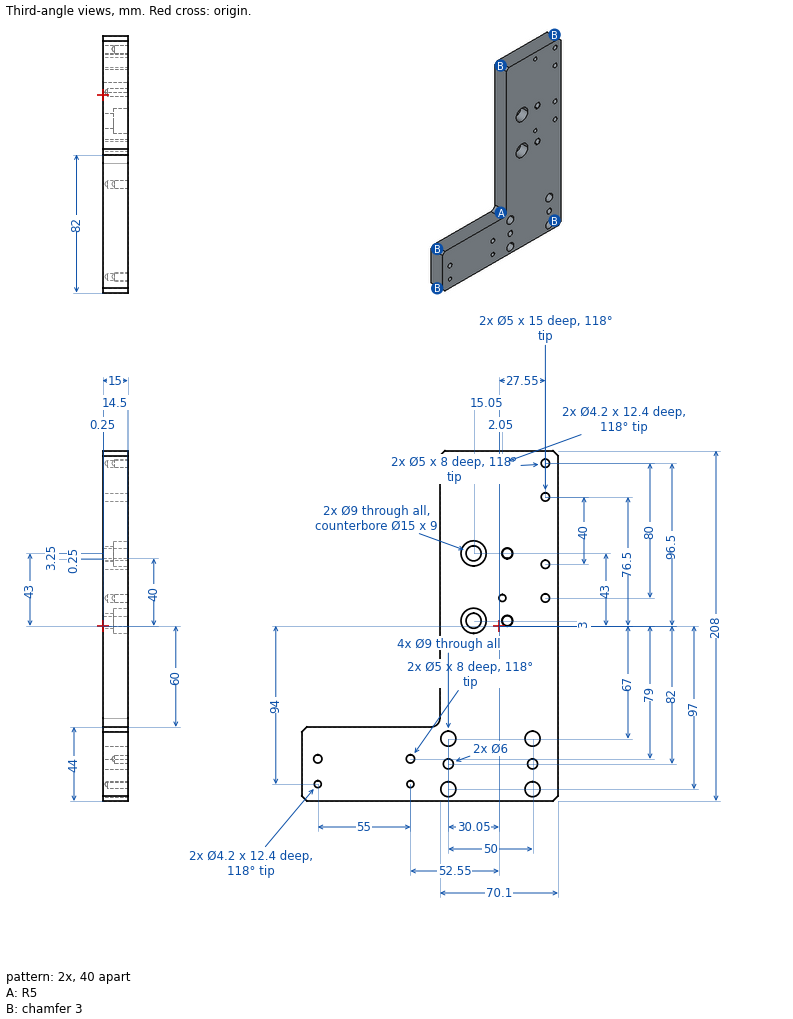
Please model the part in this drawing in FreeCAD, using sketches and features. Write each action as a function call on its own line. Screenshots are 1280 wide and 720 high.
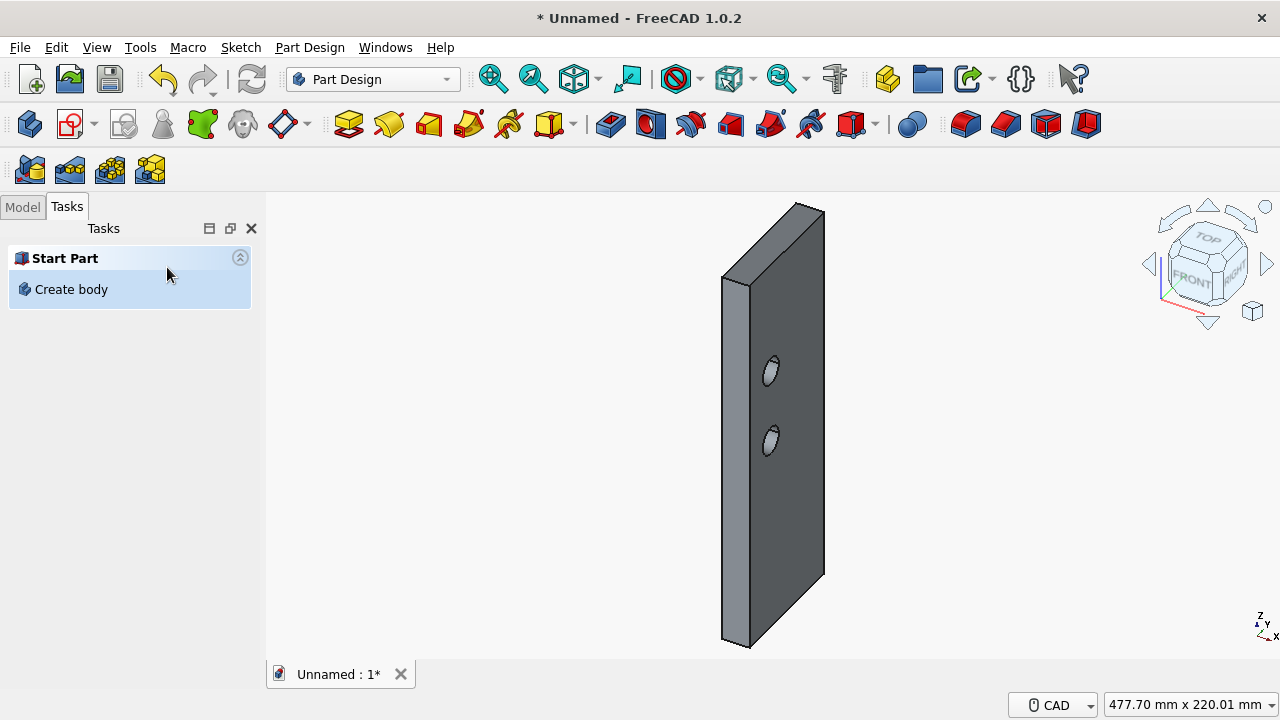
click(23, 206)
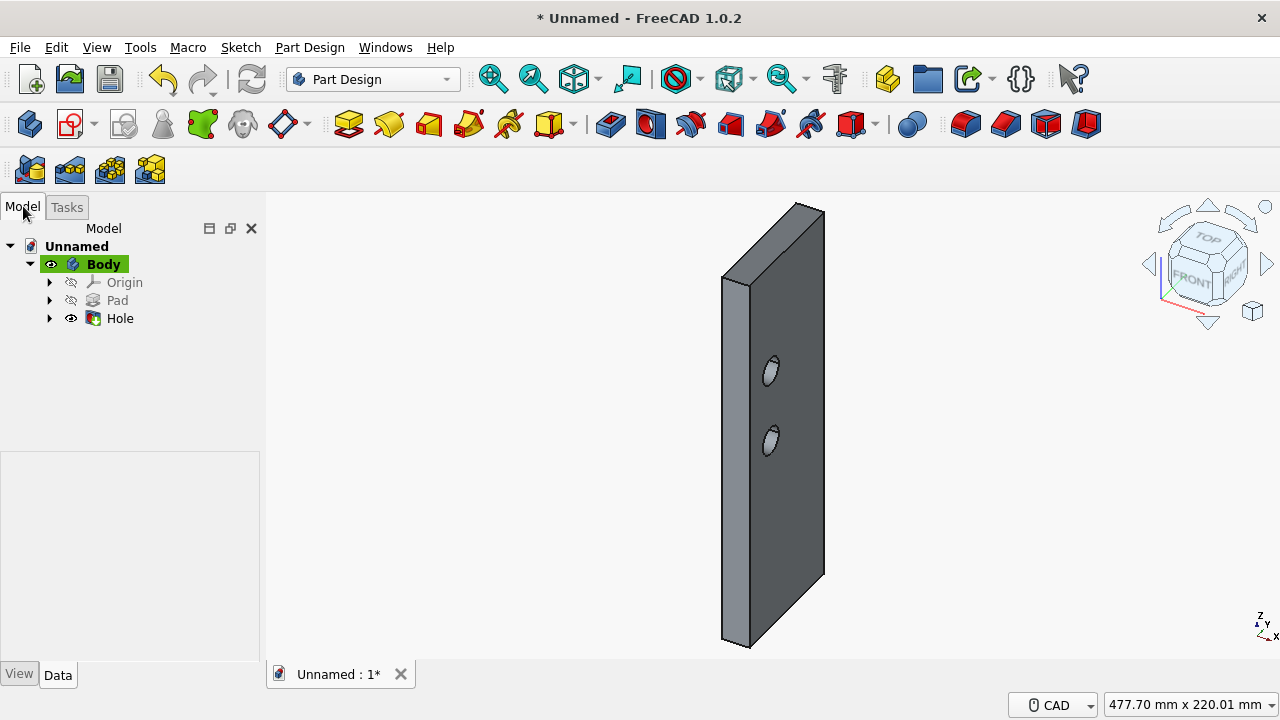
click(50, 282)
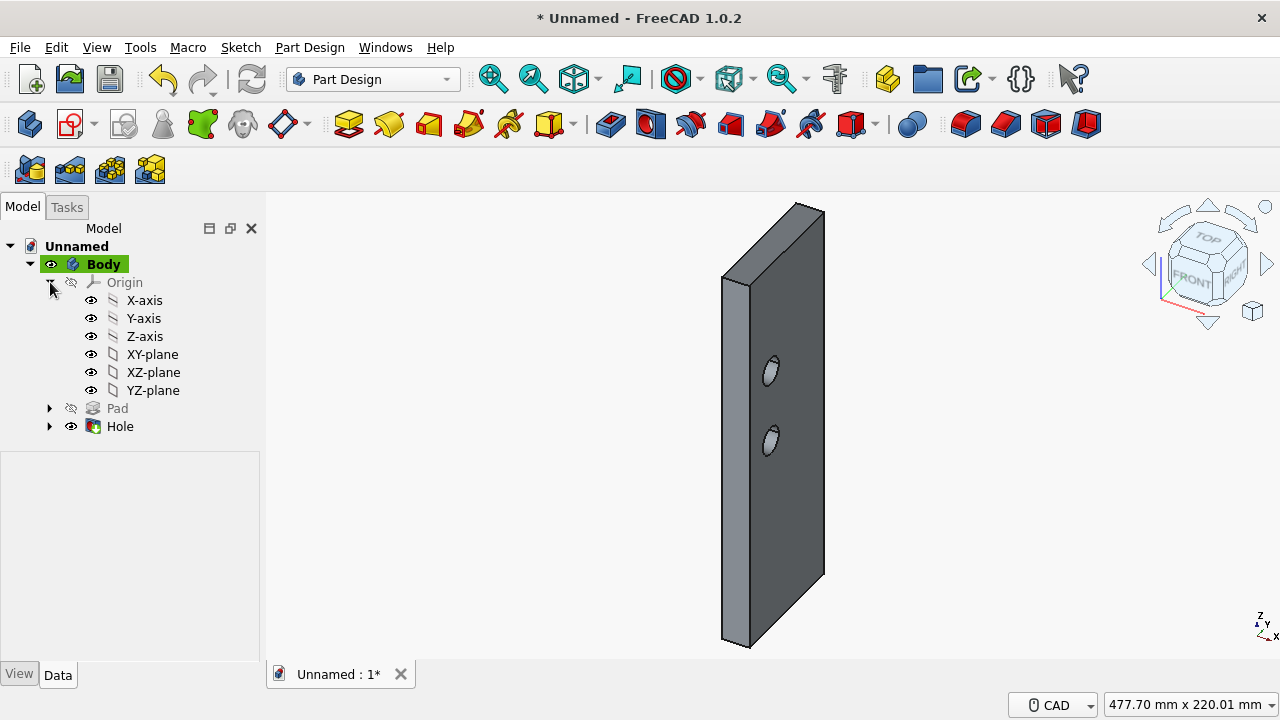
click(136, 372)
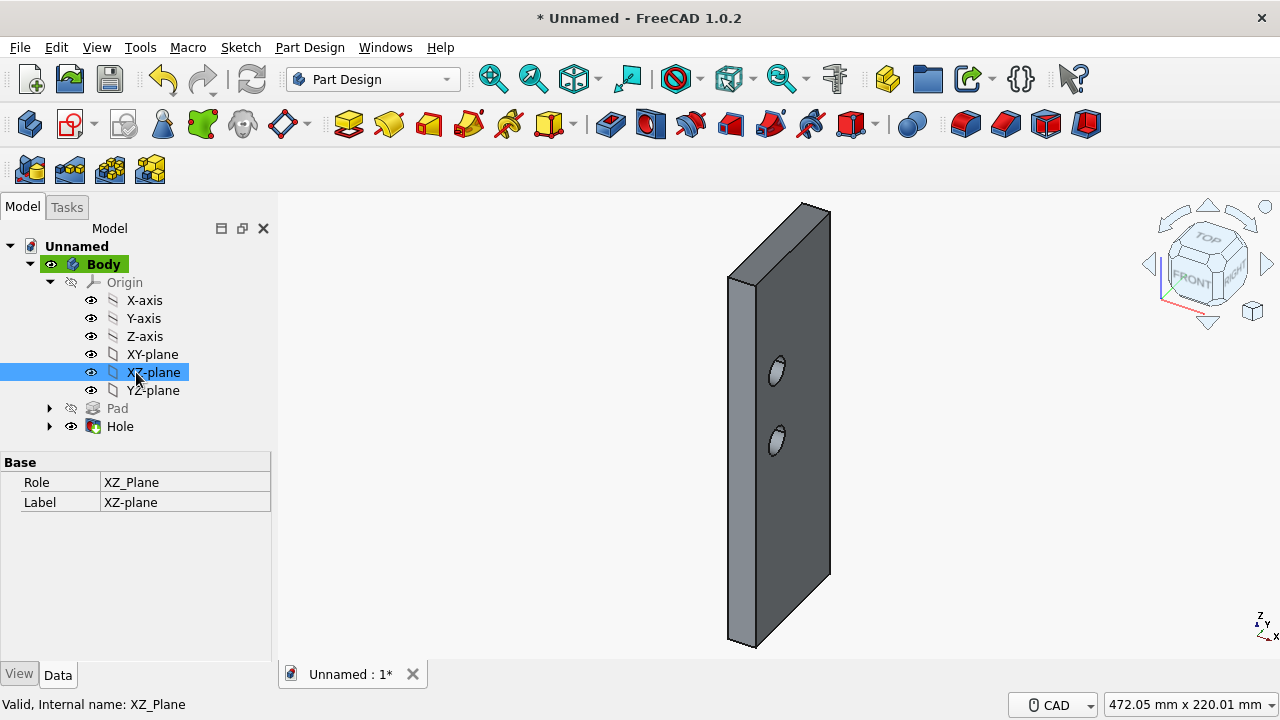
click(284, 124)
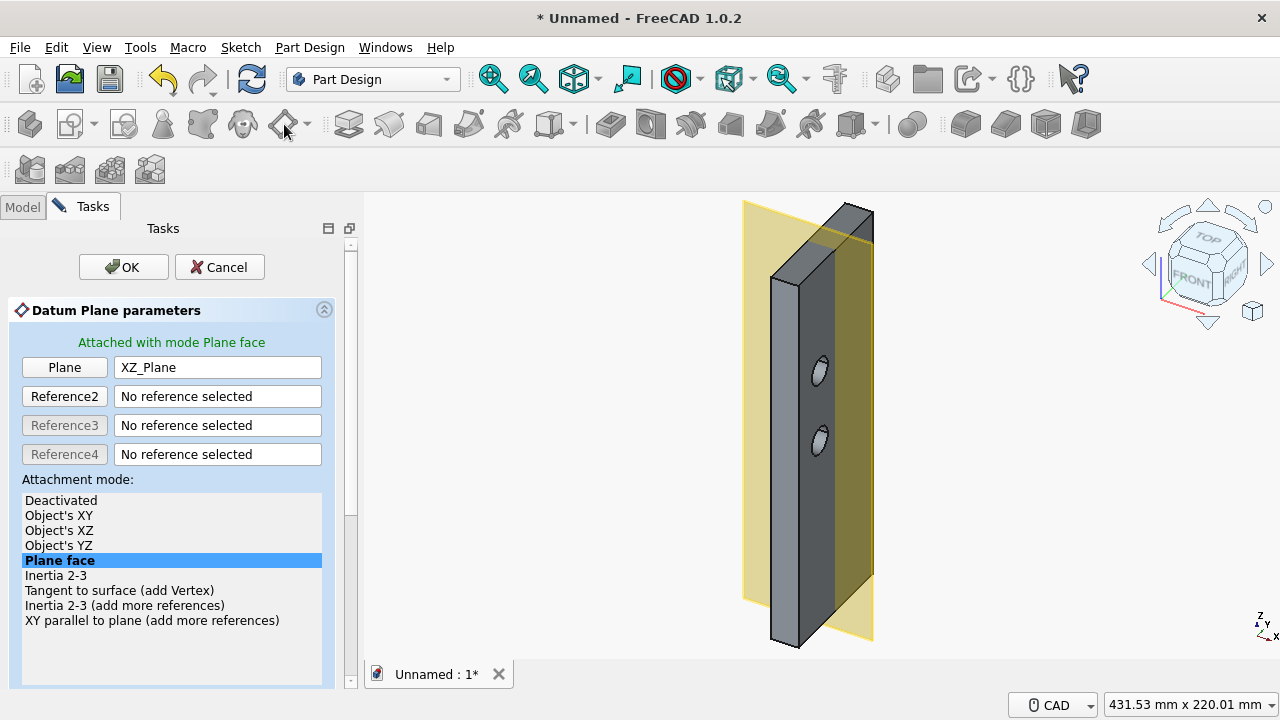
scroll(351, 463, down, 3)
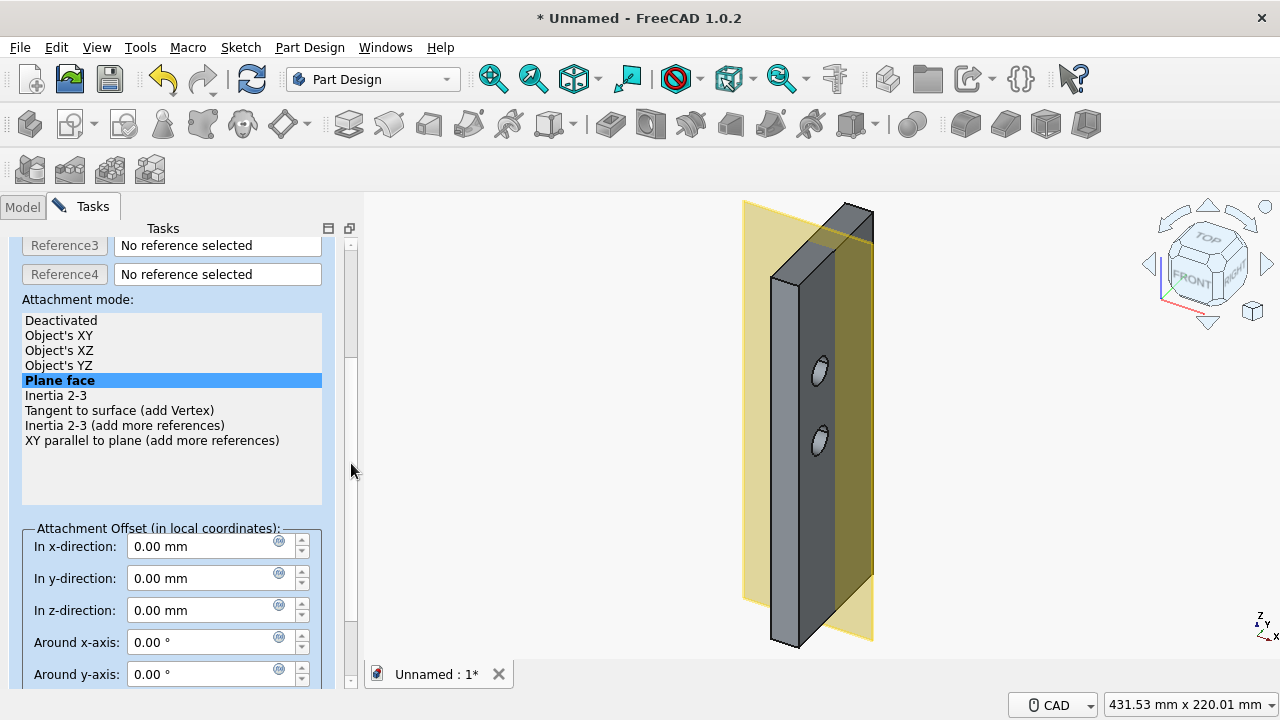
triple_click(210, 610)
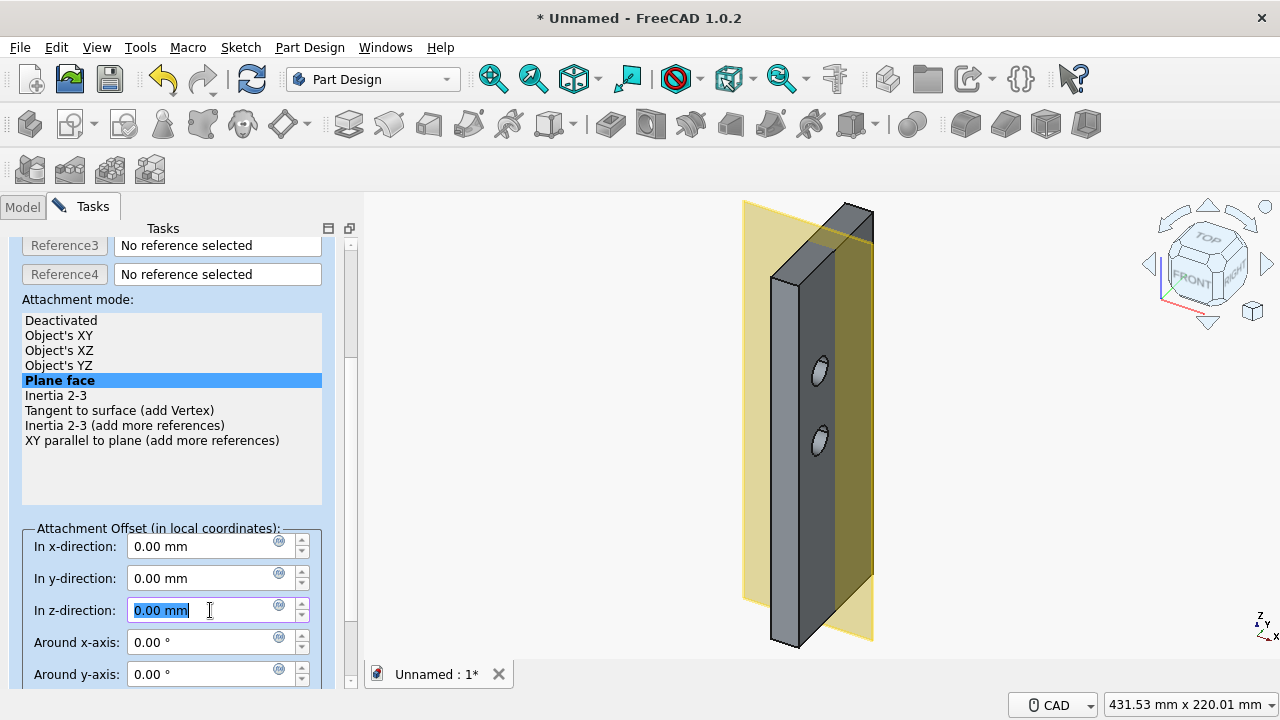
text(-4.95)
key(Tab)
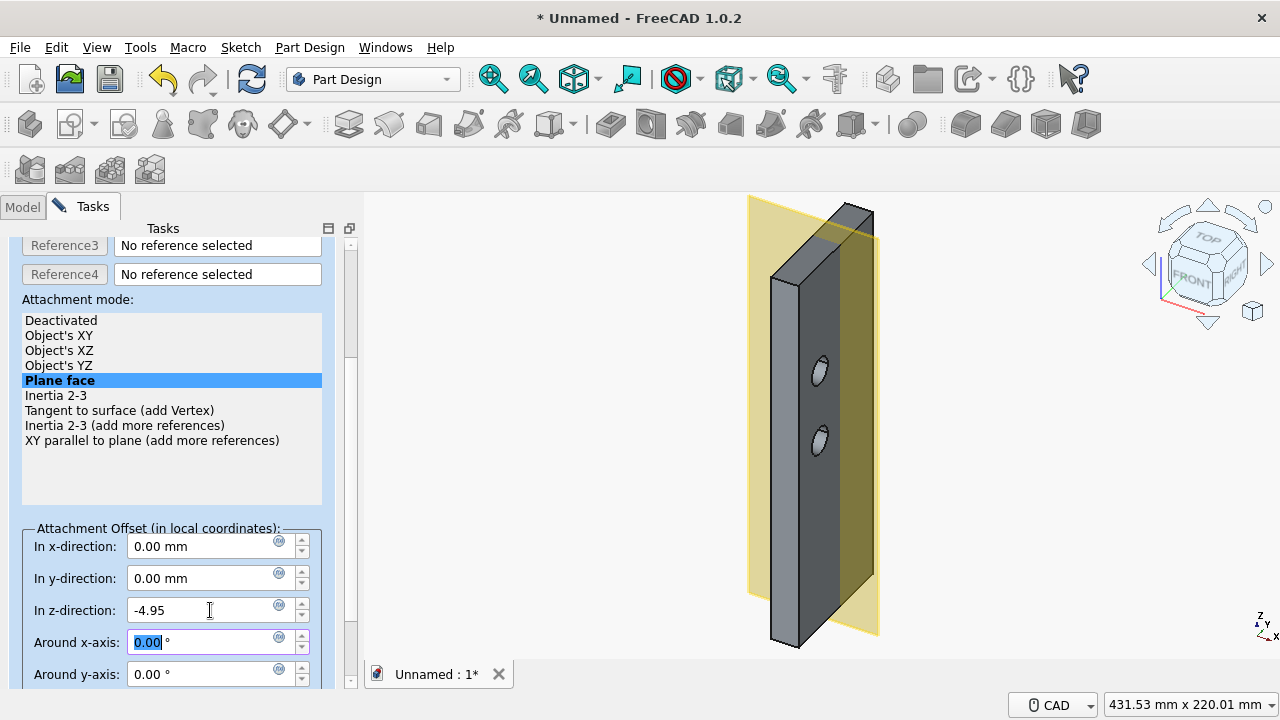
scroll(351, 463, up, 4)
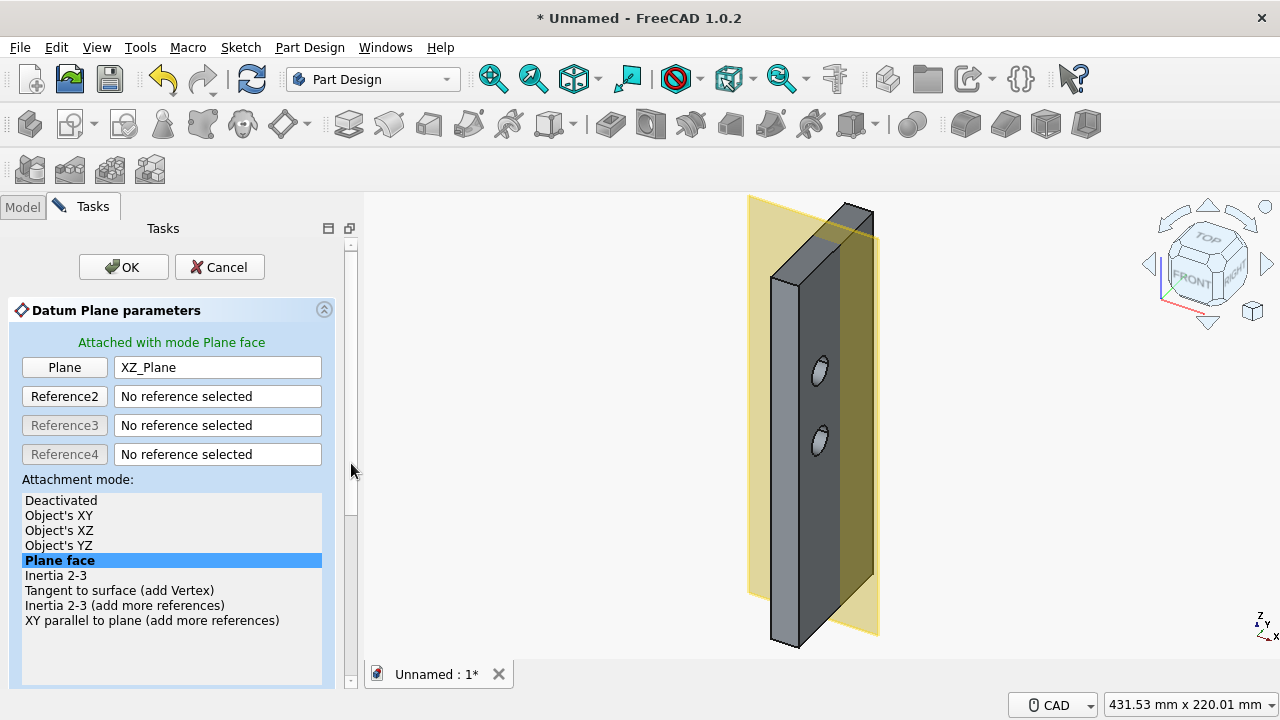
click(124, 267)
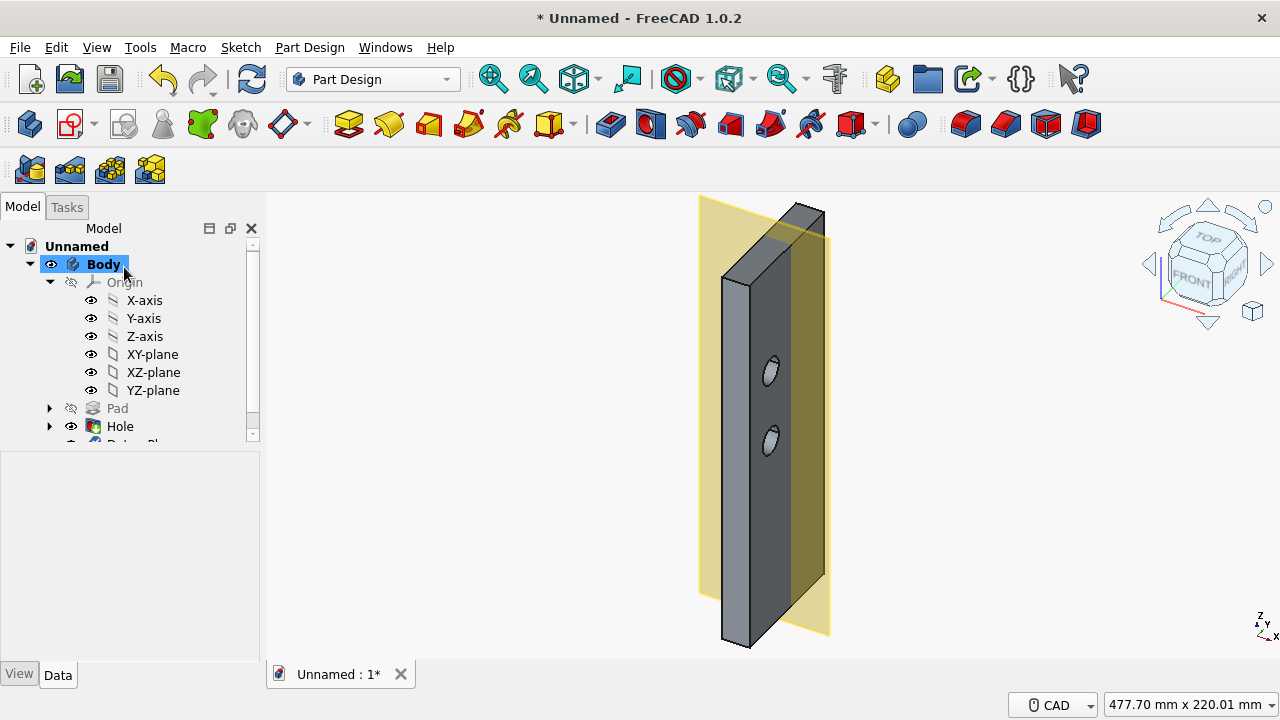
scroll(100, 332, down, 3)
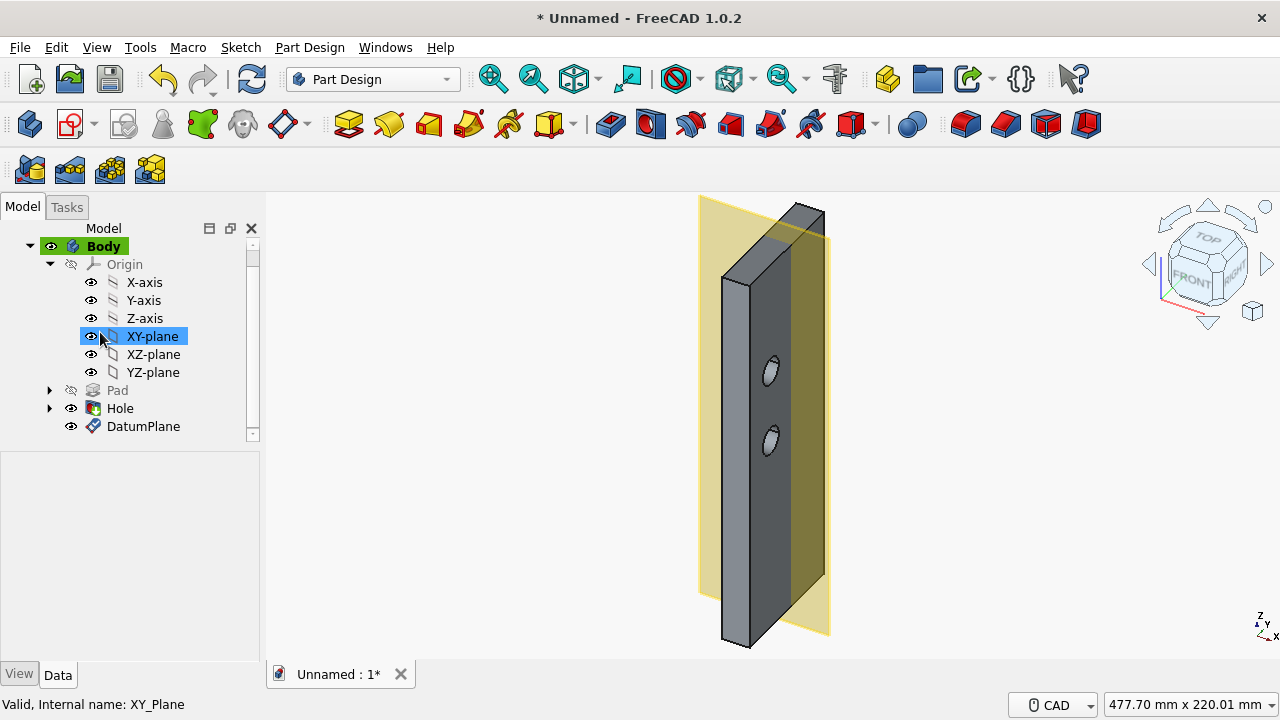
click(116, 426)